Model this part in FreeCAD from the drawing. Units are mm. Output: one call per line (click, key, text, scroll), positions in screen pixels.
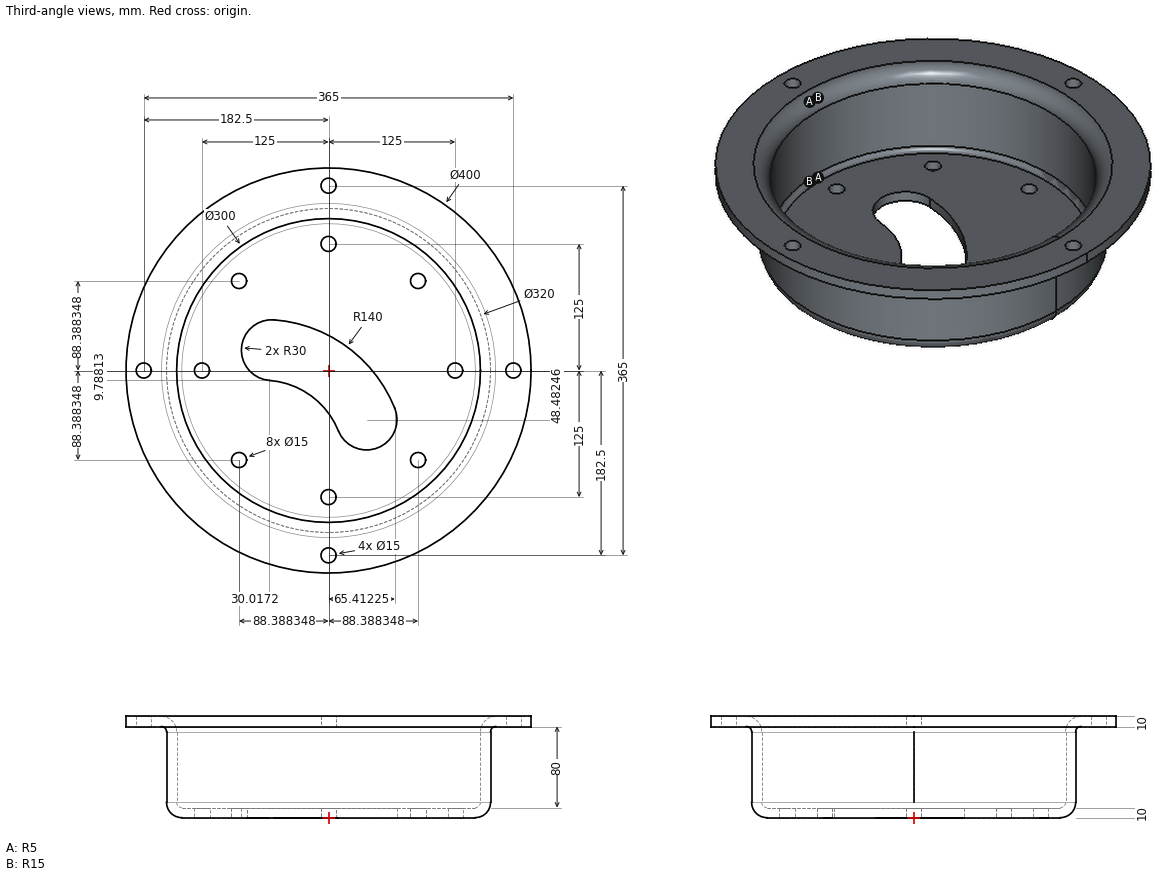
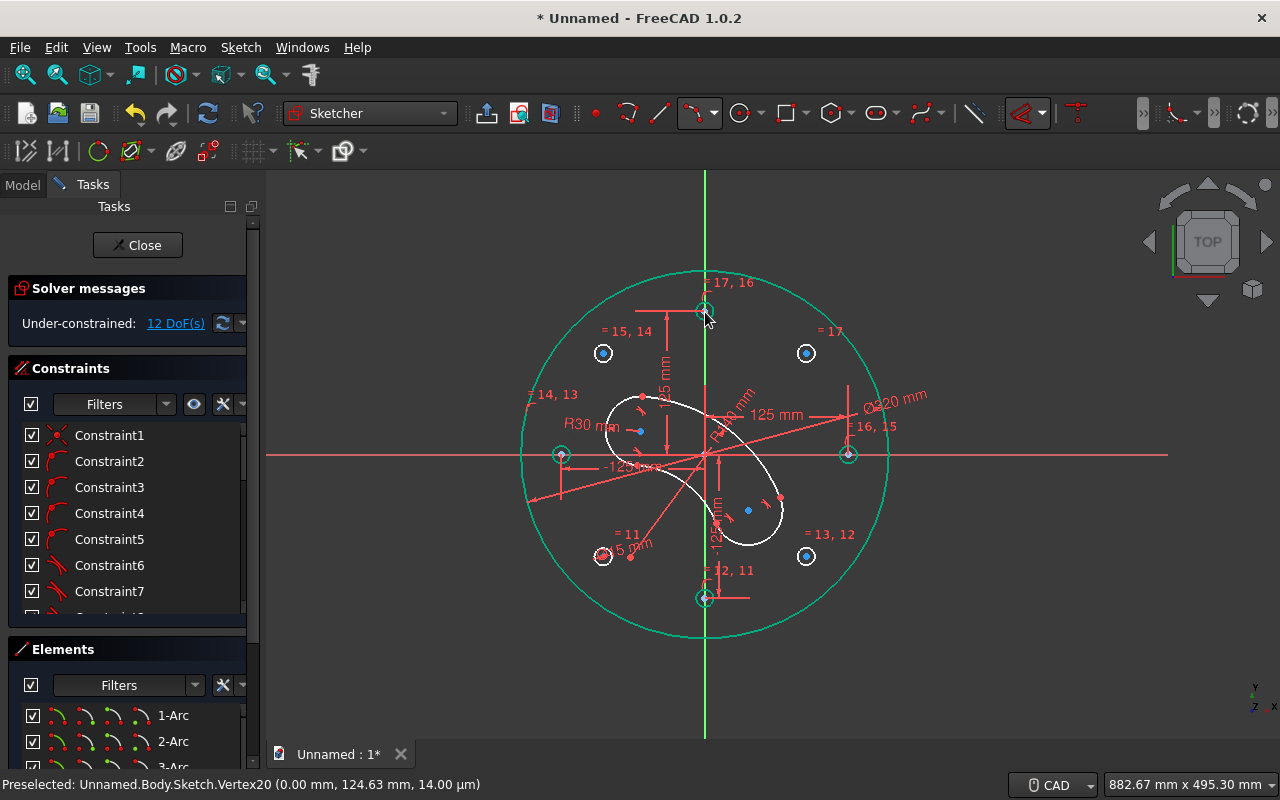
scroll(638, 465, up, 7)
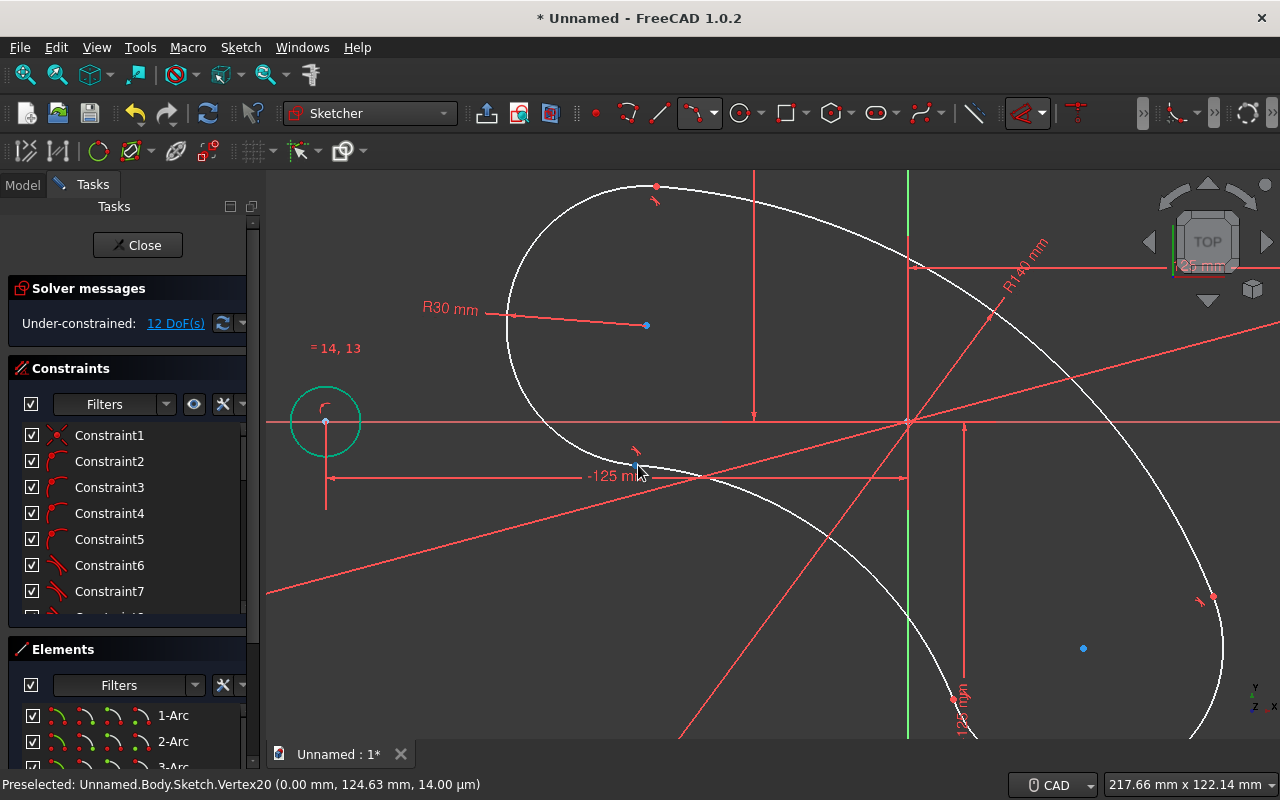
click(636, 465)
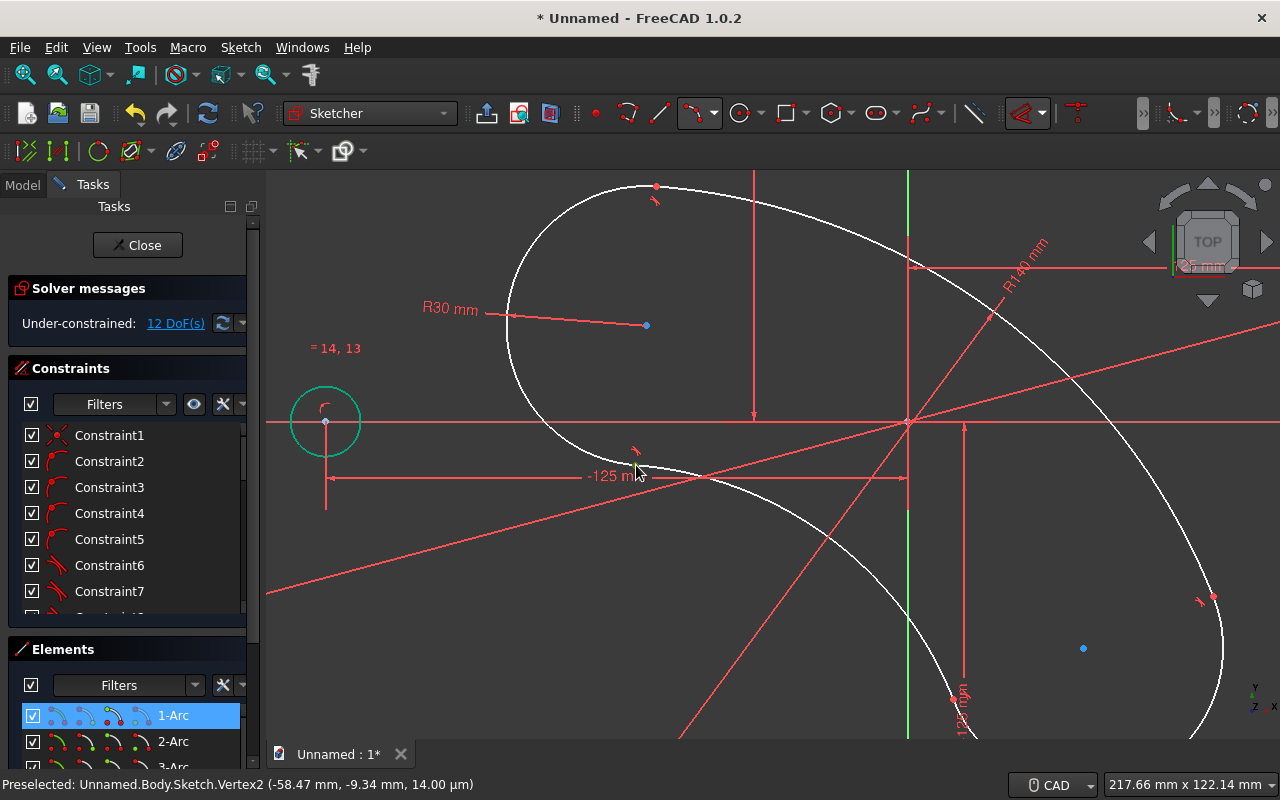
click(1044, 114)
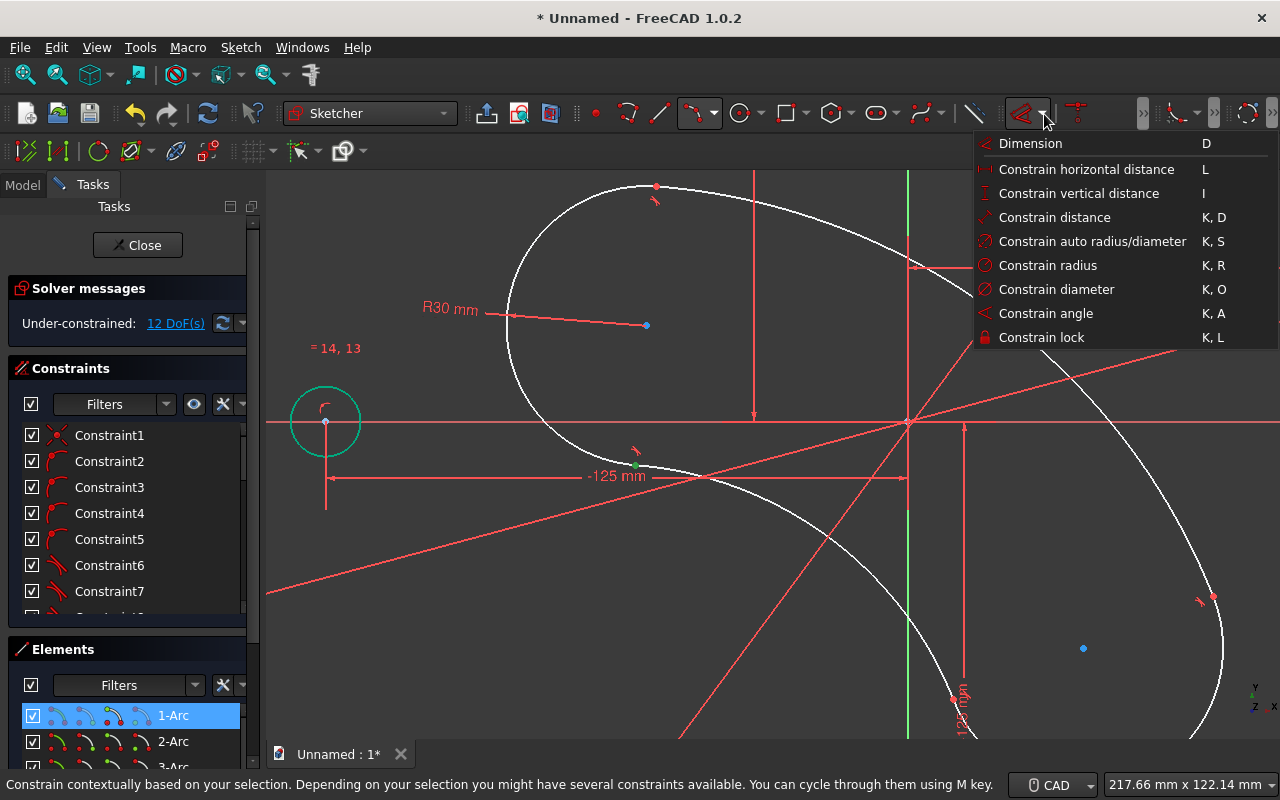
click(1126, 193)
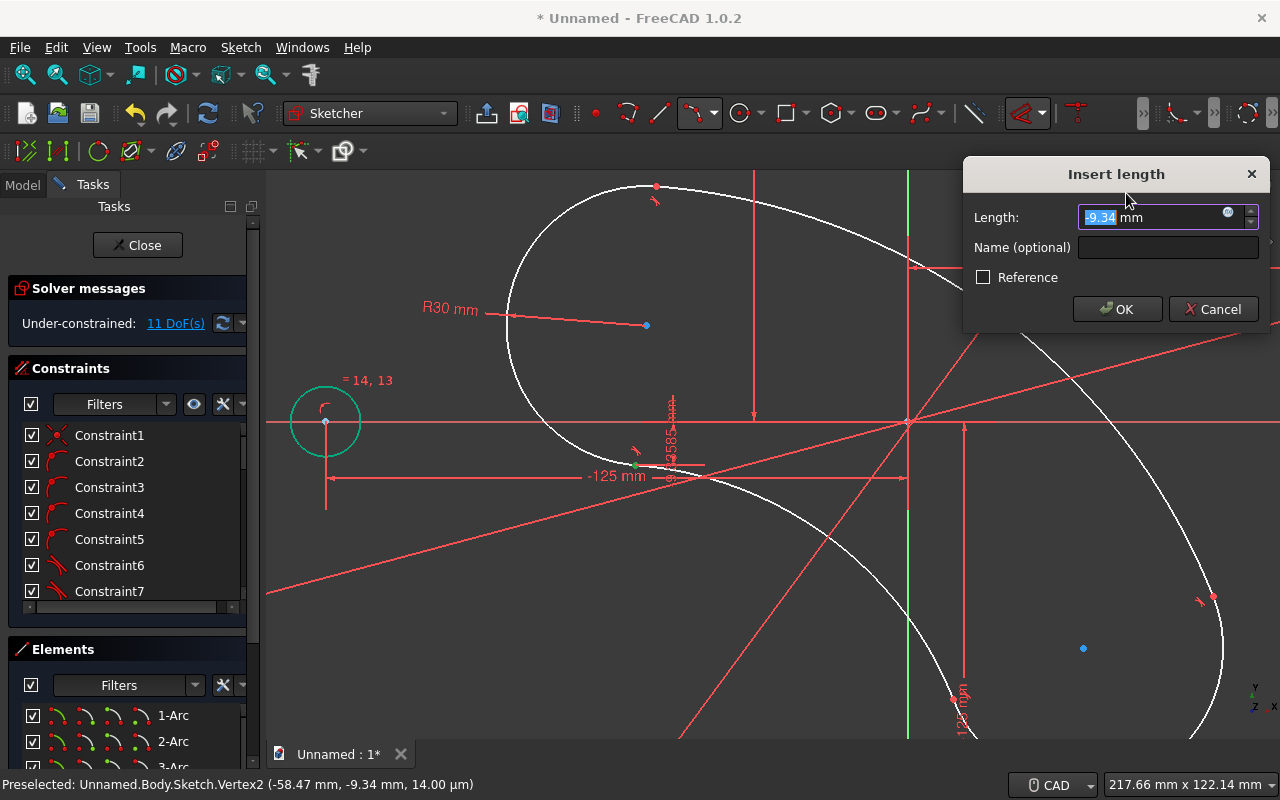
text(-9.78813)
key(Return)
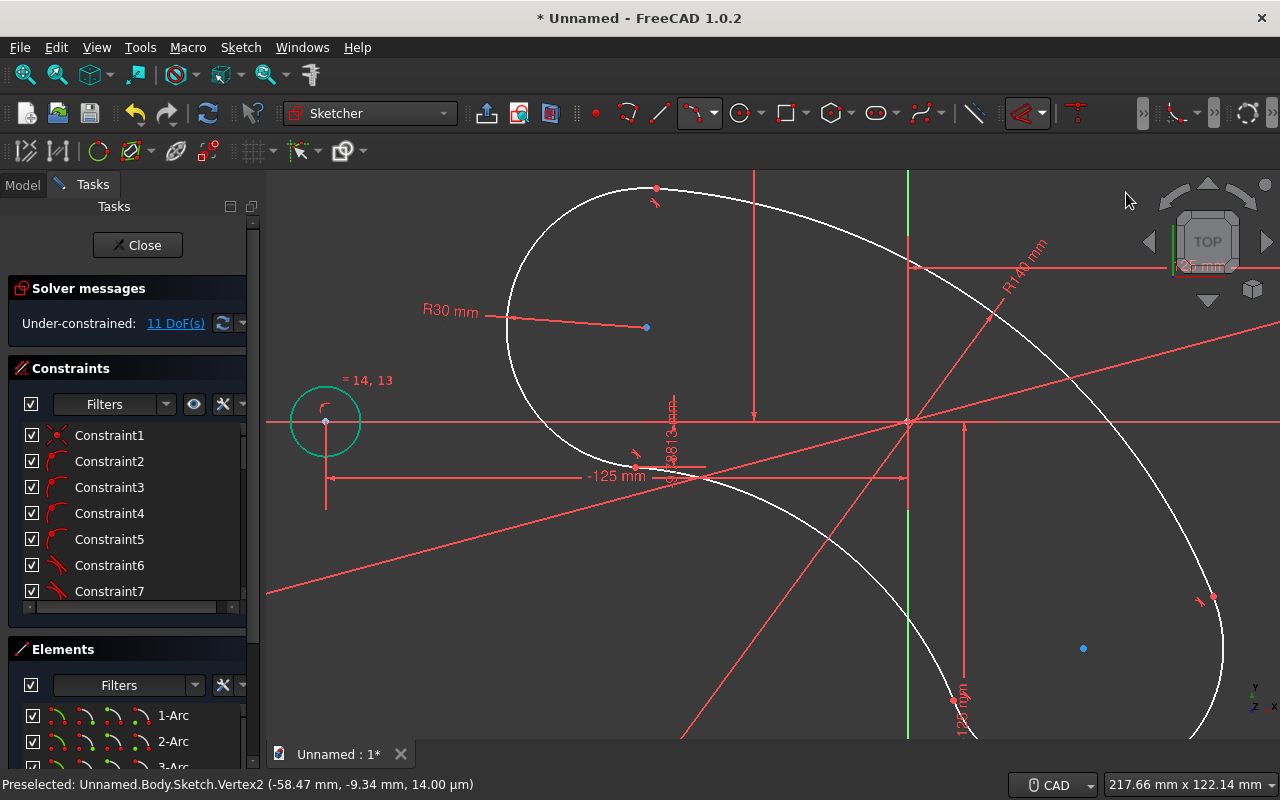
scroll(638, 465, down, 7)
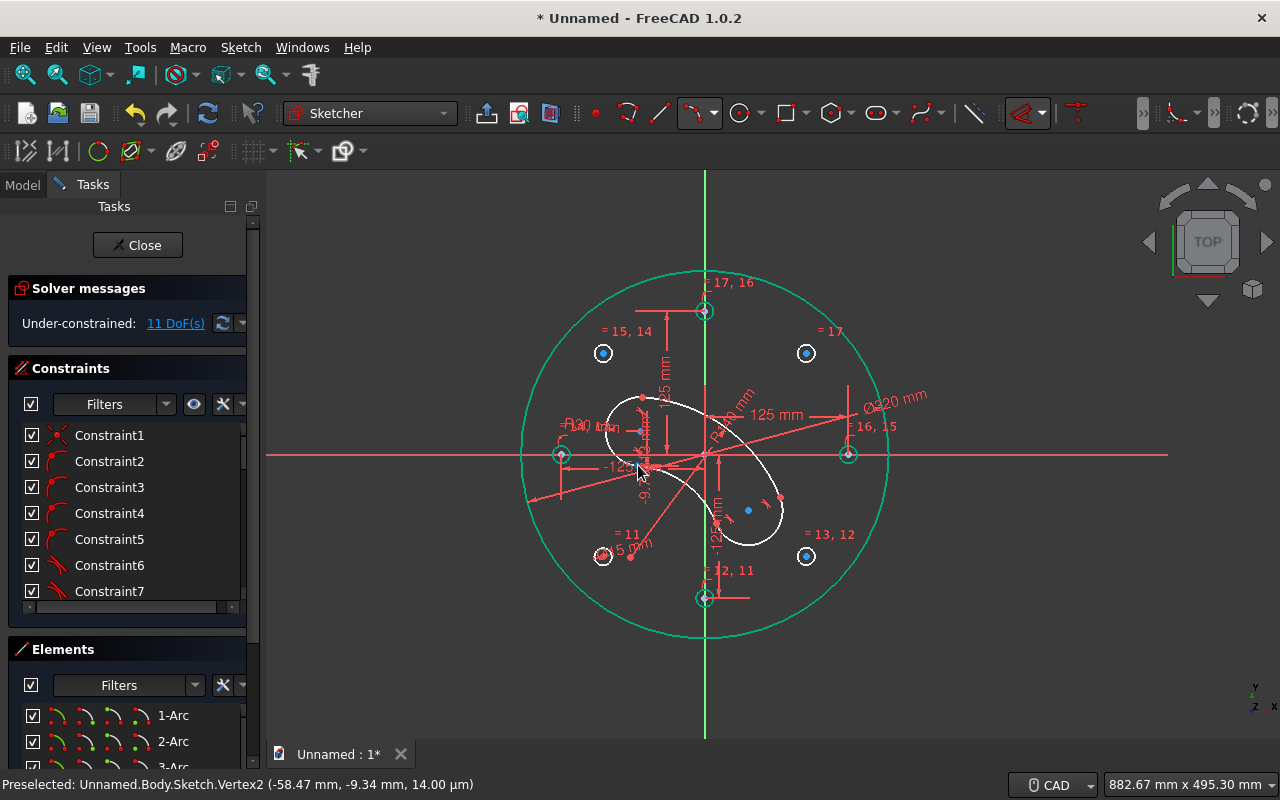
click(638, 466)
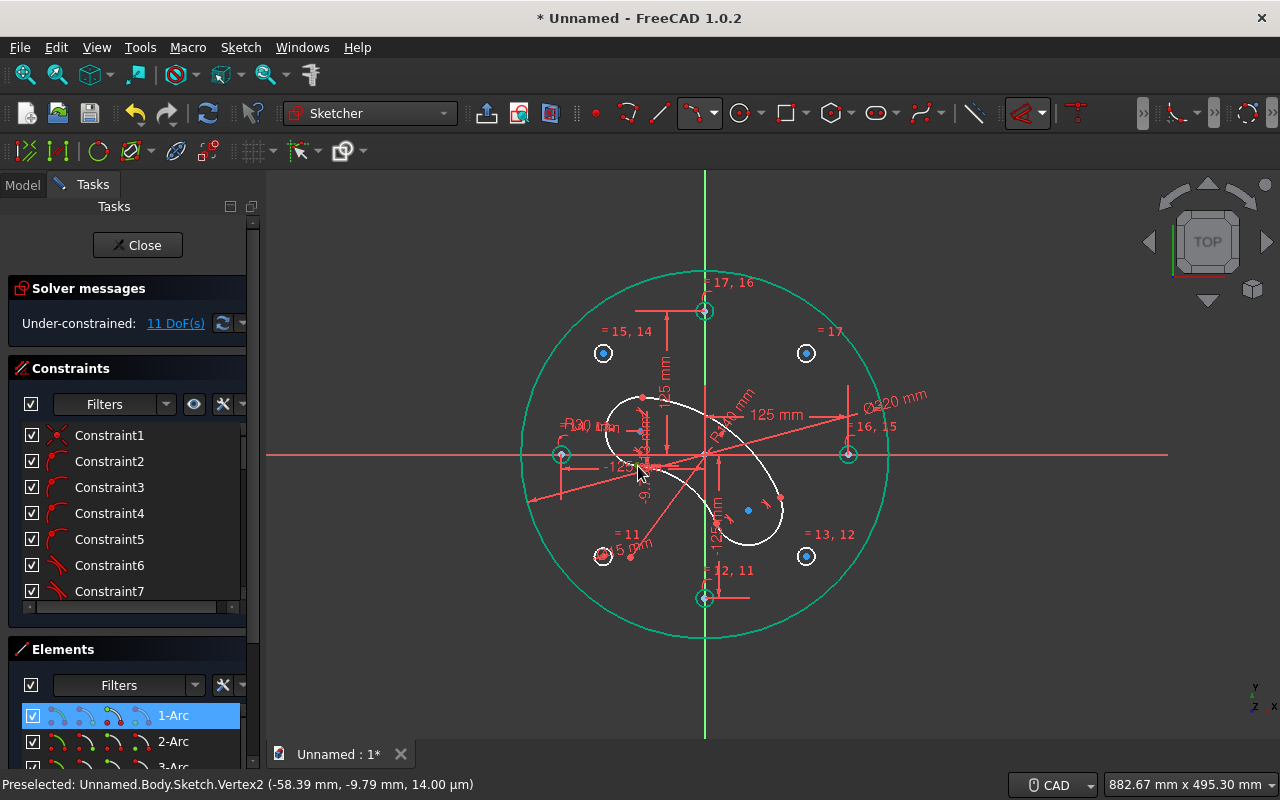
click(603, 557)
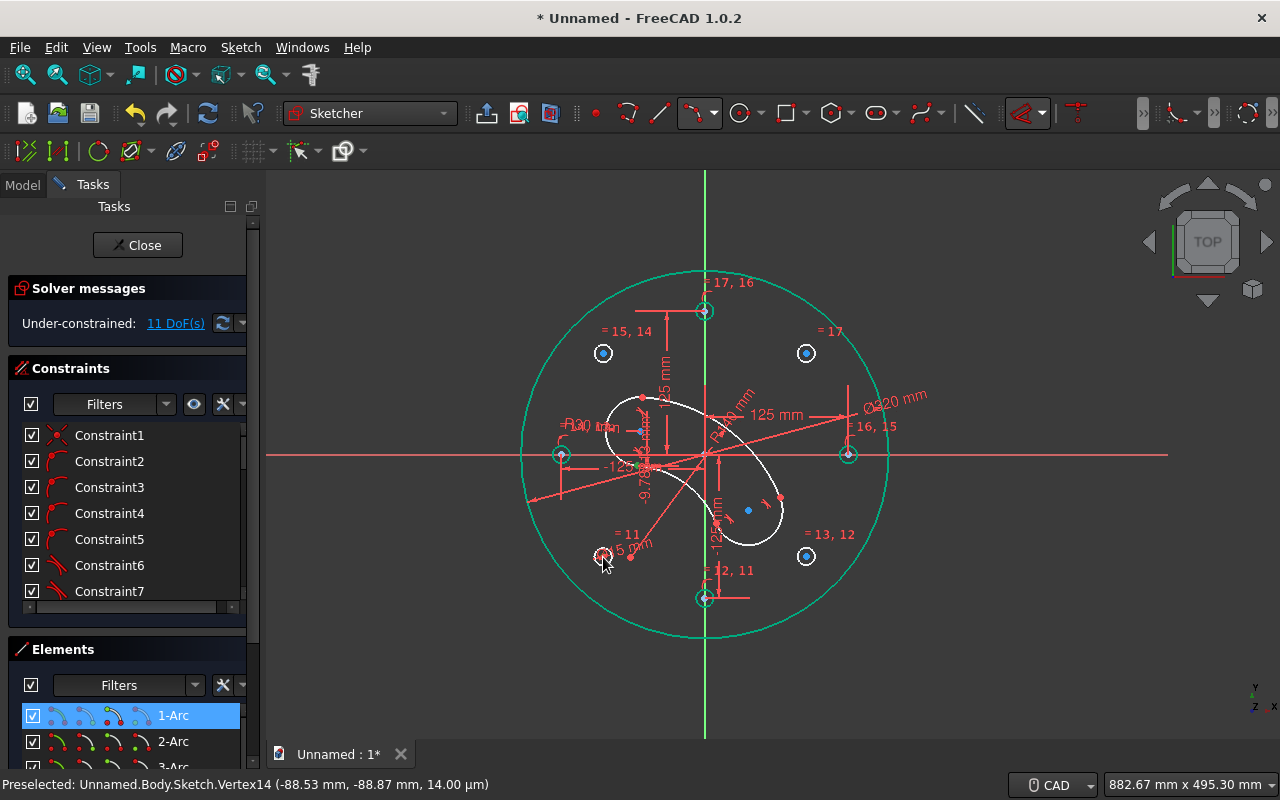
click(1044, 114)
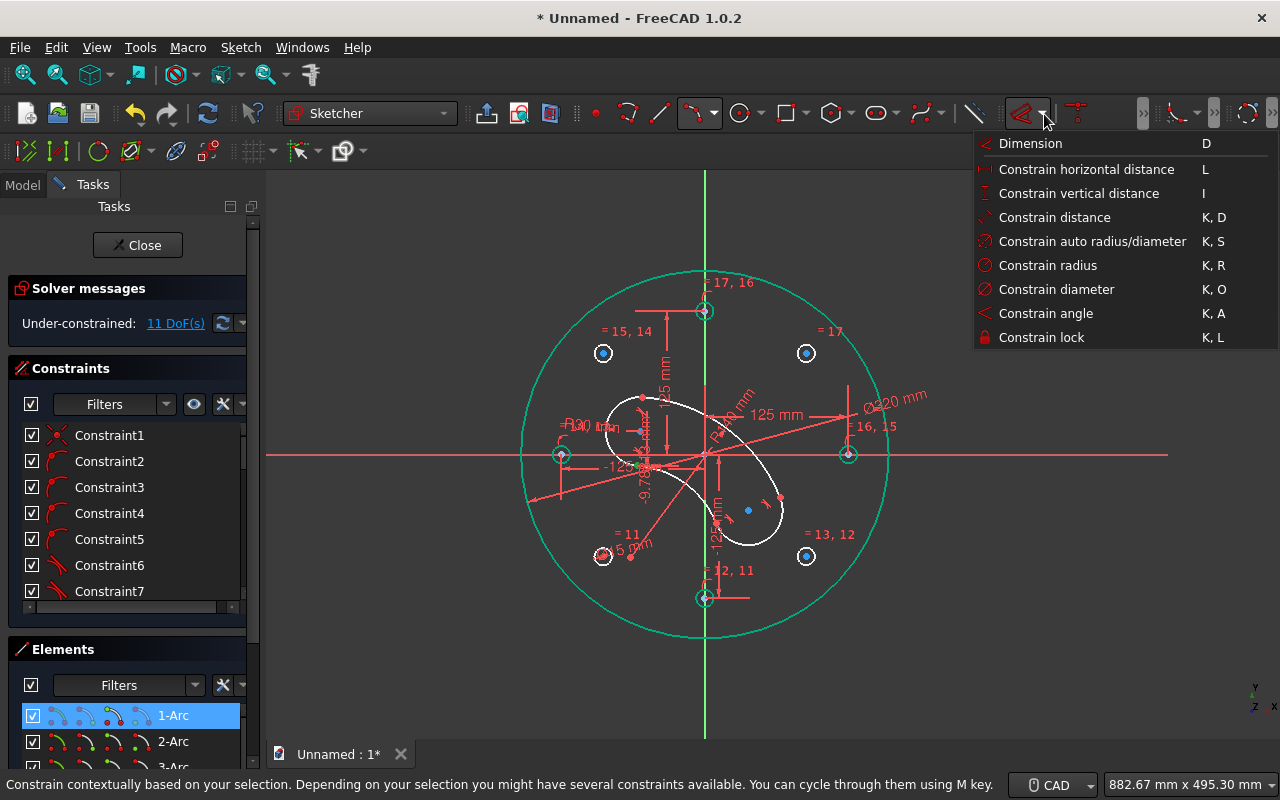
click(1126, 169)